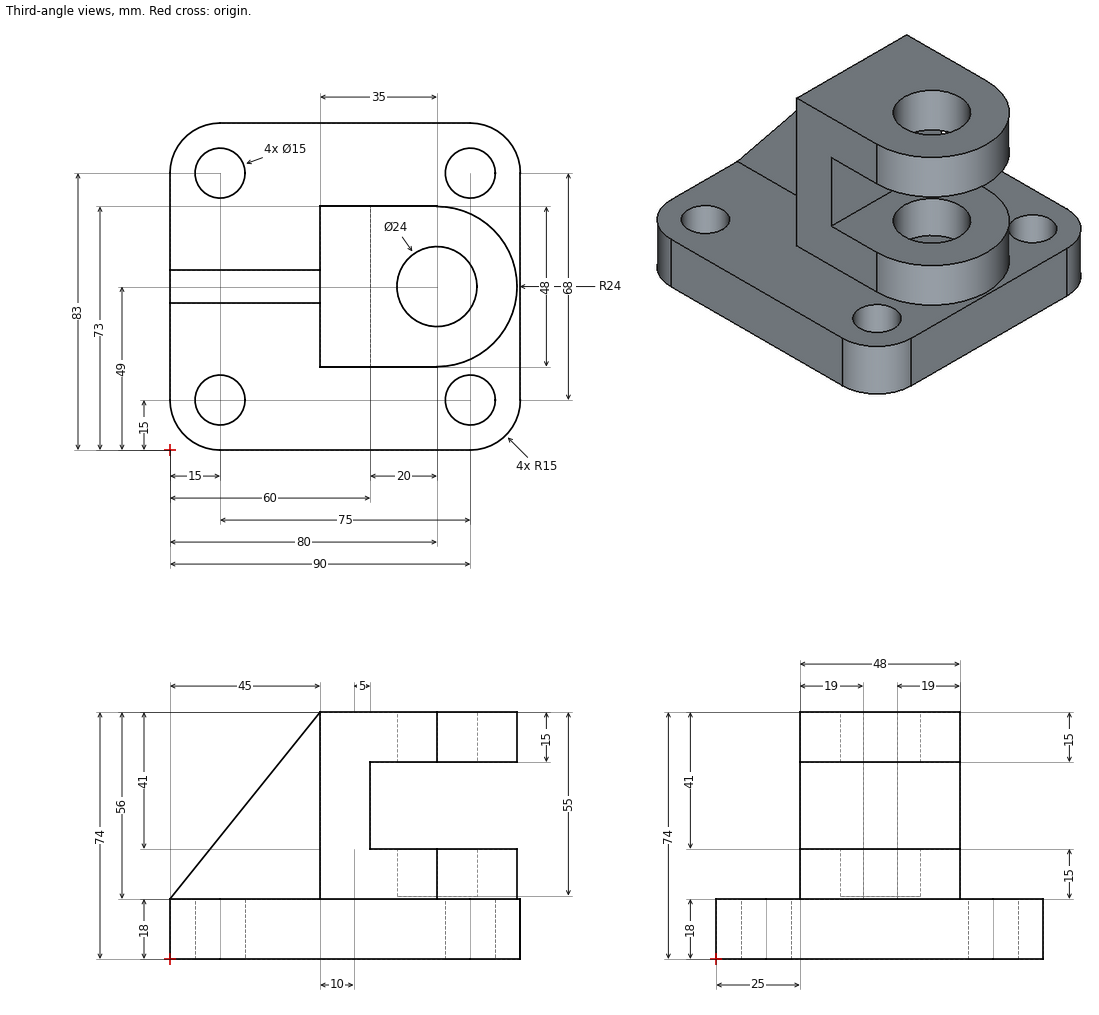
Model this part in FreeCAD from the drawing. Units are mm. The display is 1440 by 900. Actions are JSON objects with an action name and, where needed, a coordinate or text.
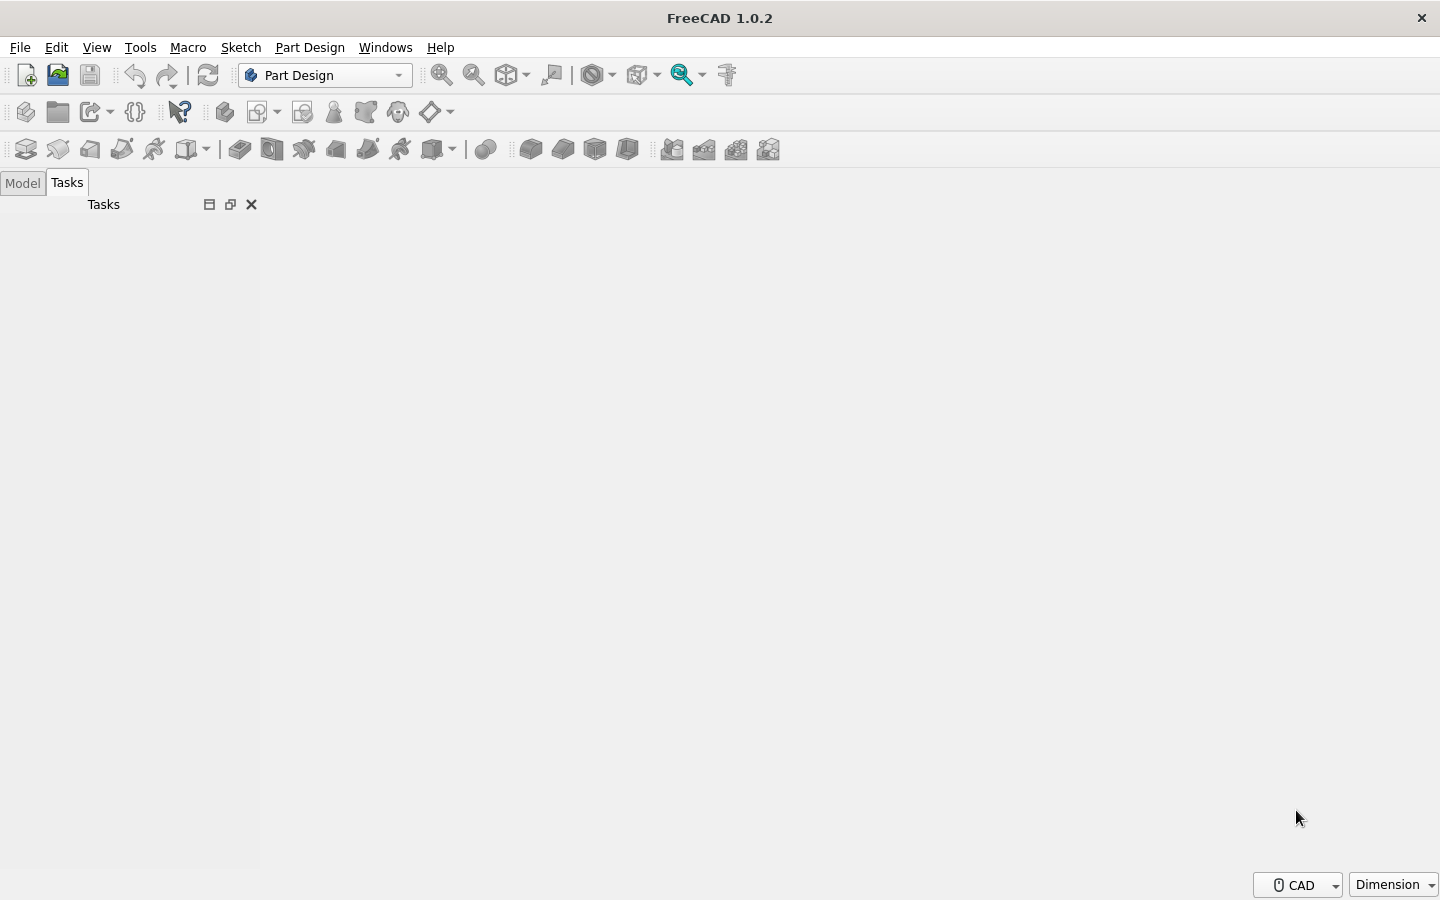
{"action": "left_click", "coordinate": [26, 76]}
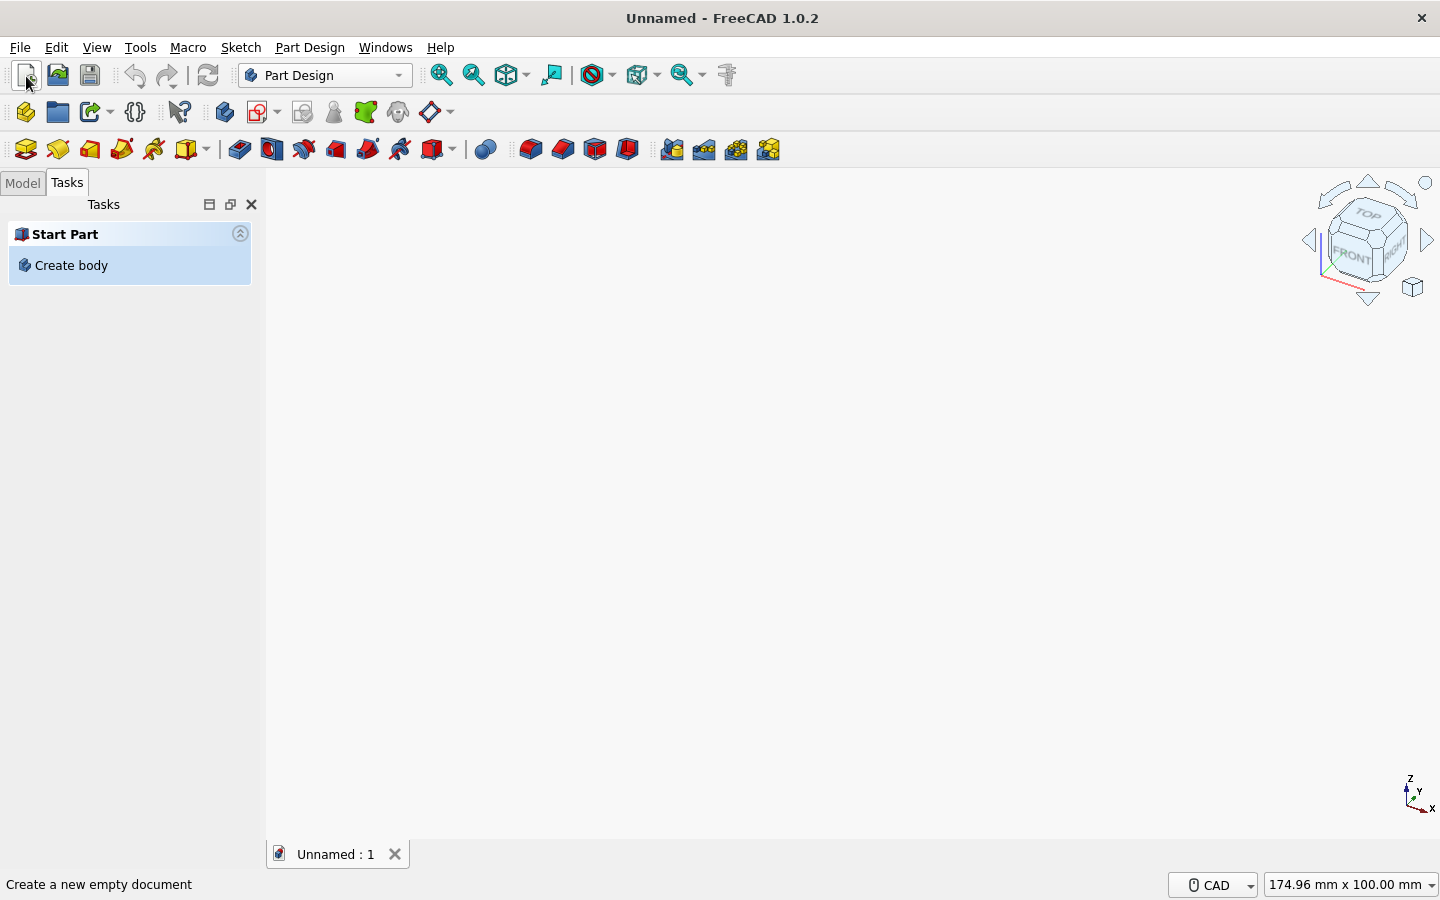
{"action": "left_click", "coordinate": [258, 112]}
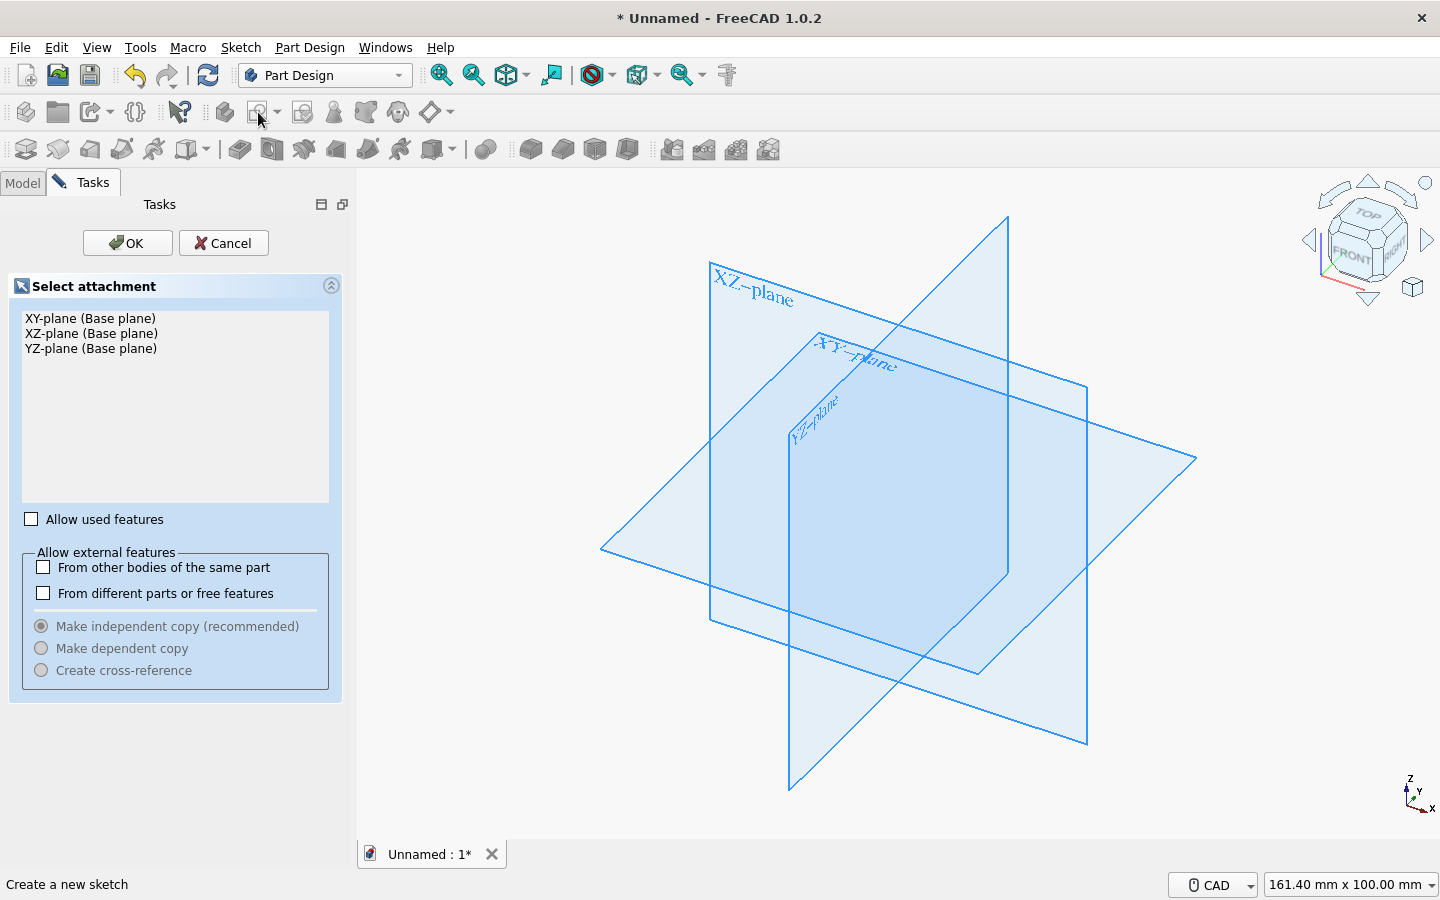
{"action": "left_click", "coordinate": [82, 318]}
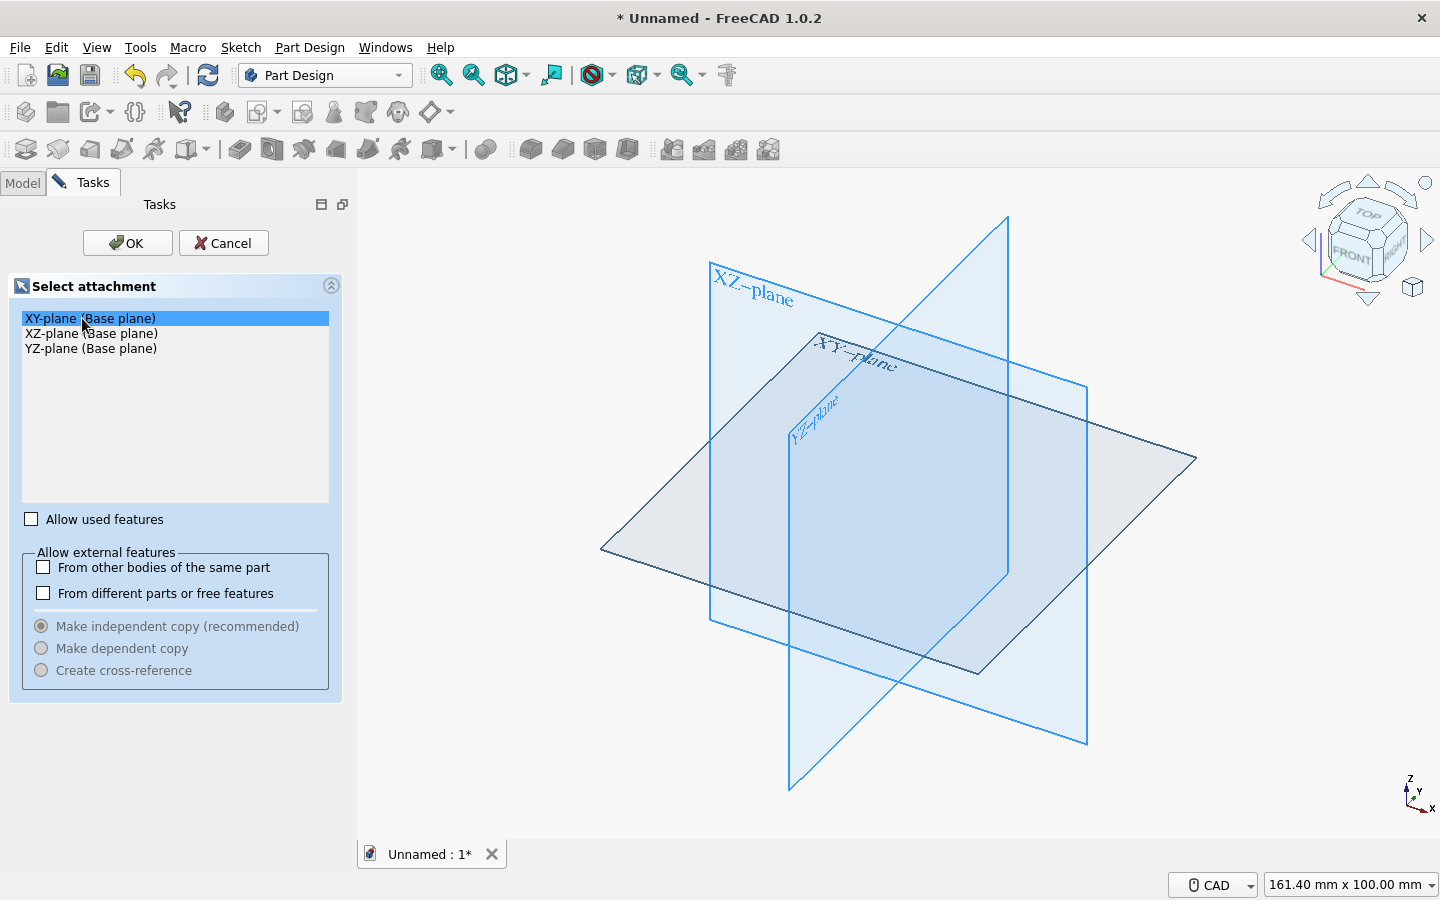
{"action": "left_click", "coordinate": [128, 243]}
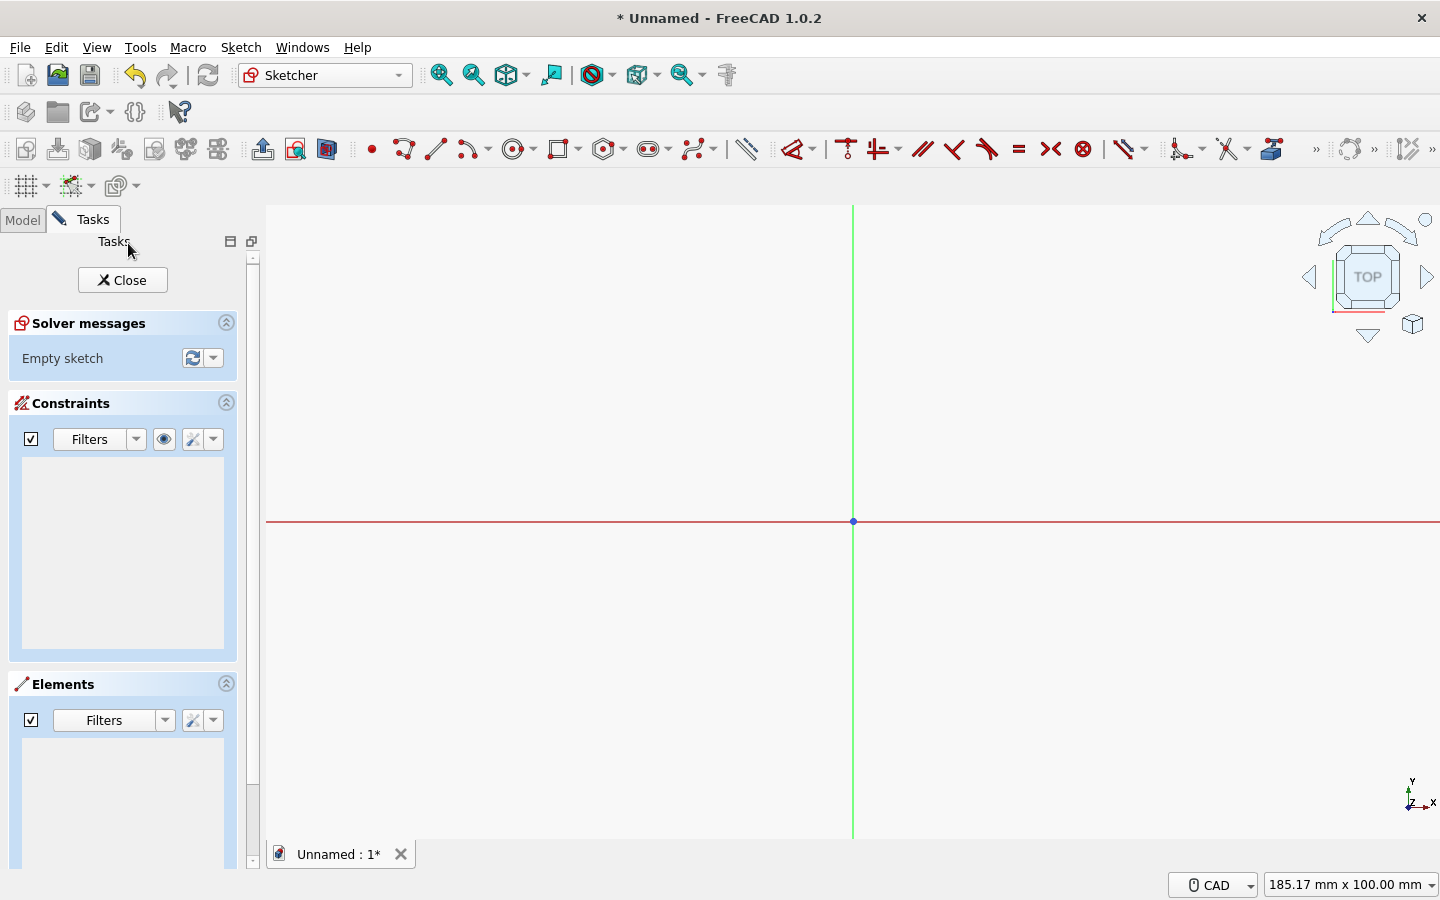
{"action": "scroll", "coordinate": [296, 811], "scroll_direction": "down", "scroll_amount": 3}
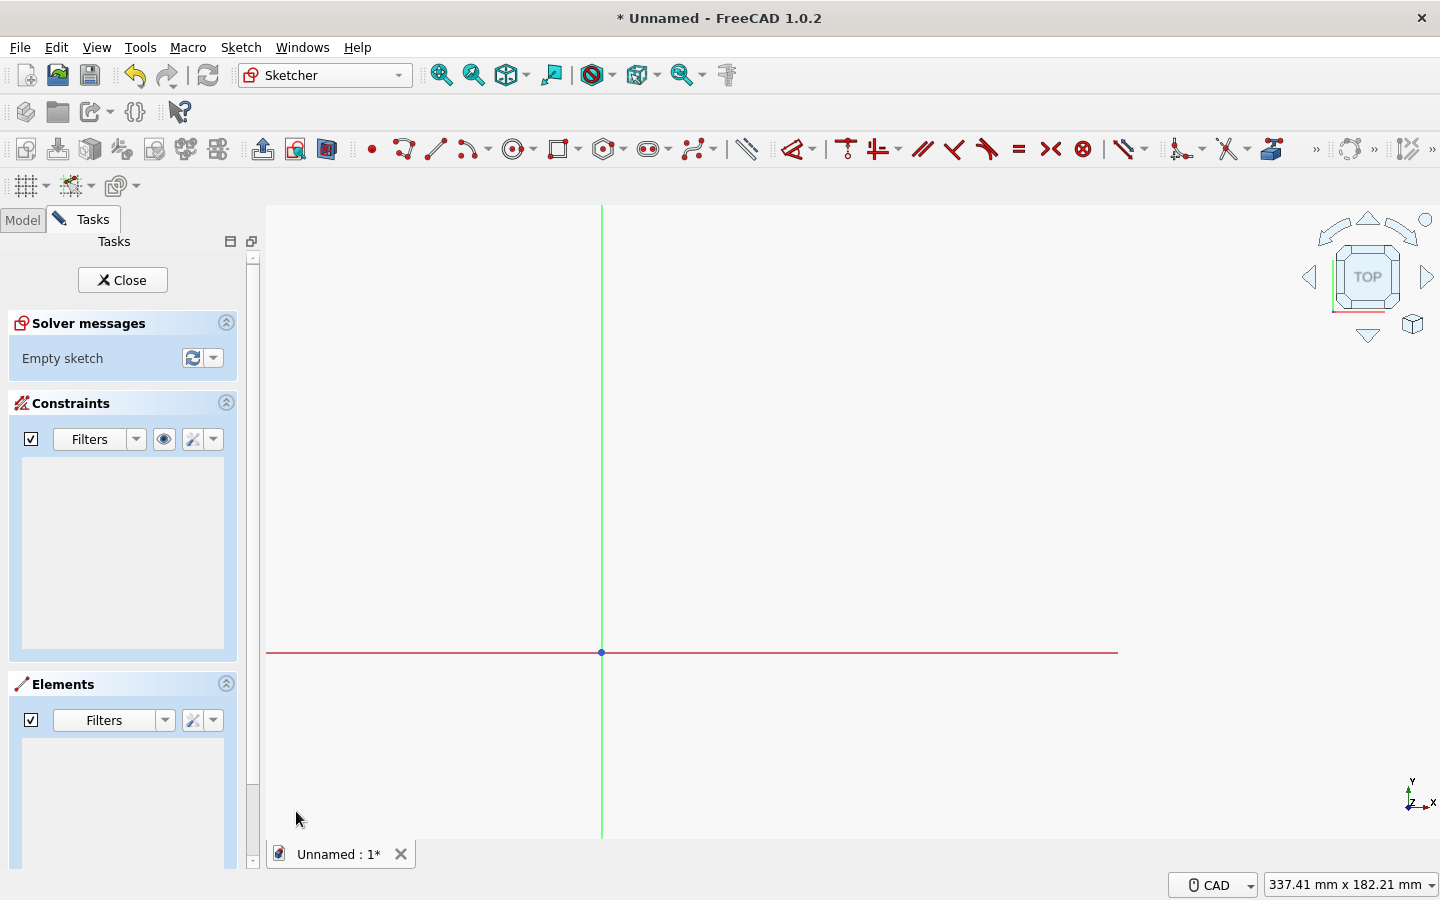
{"action": "left_click", "coordinate": [436, 150]}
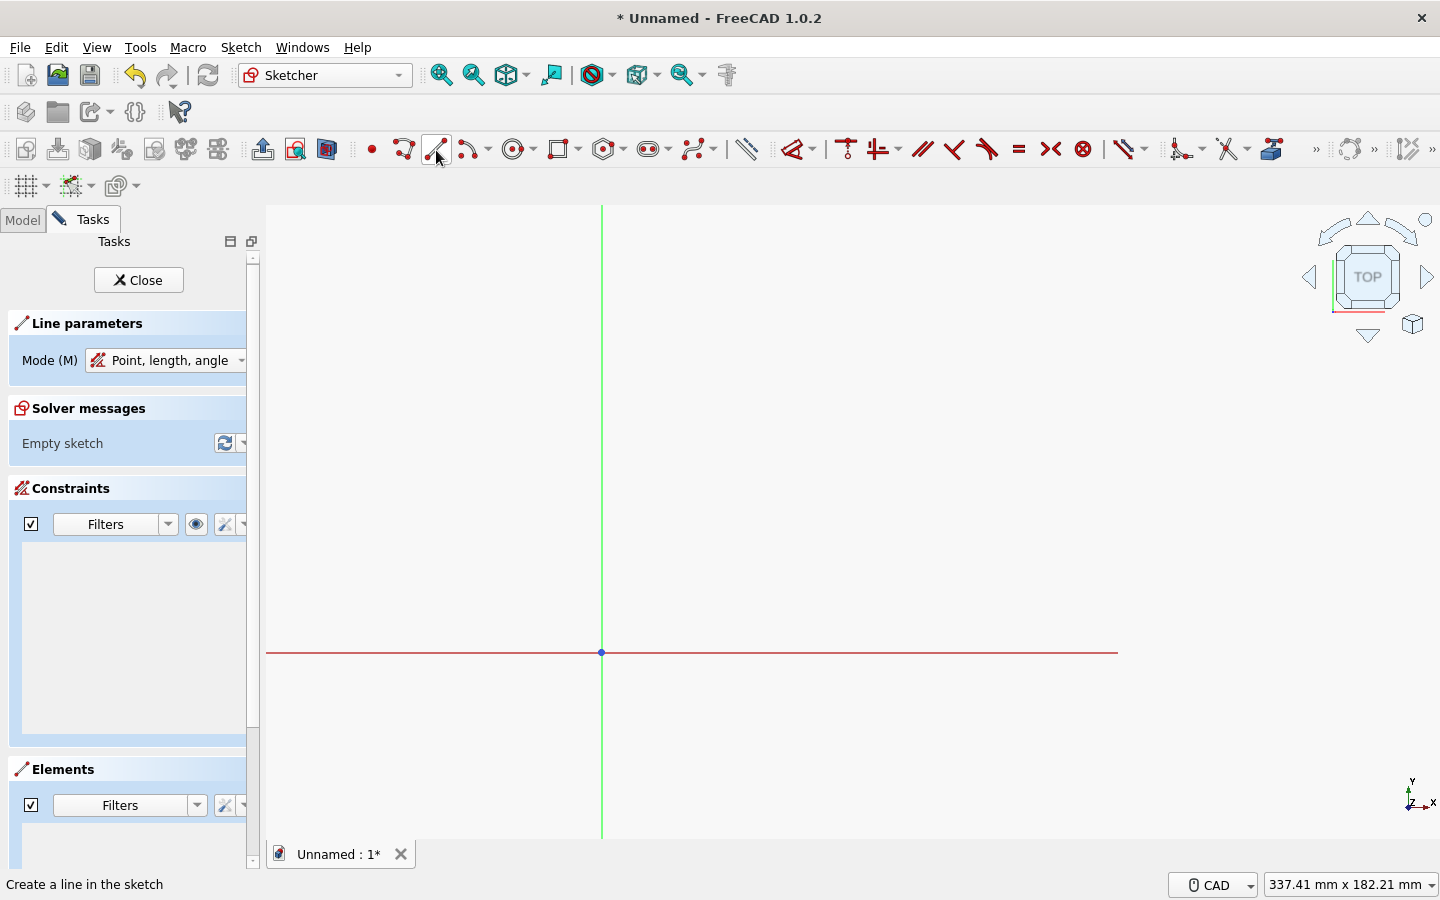
{"action": "left_click", "coordinate": [654, 653]}
{"action": "left_click", "coordinate": [915, 644]}